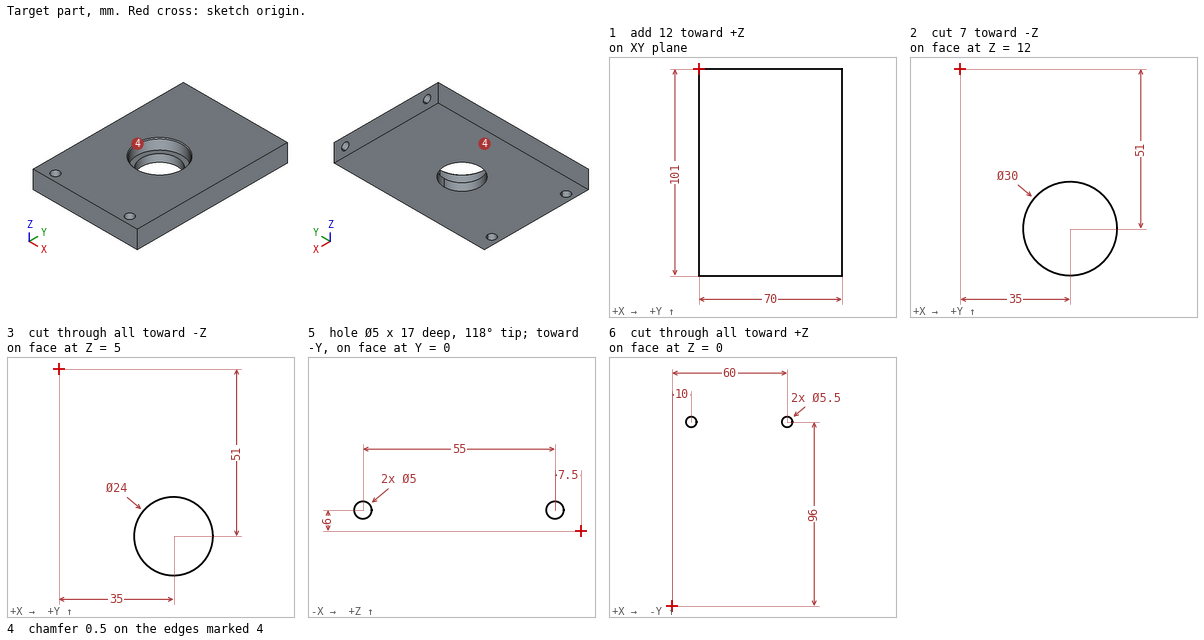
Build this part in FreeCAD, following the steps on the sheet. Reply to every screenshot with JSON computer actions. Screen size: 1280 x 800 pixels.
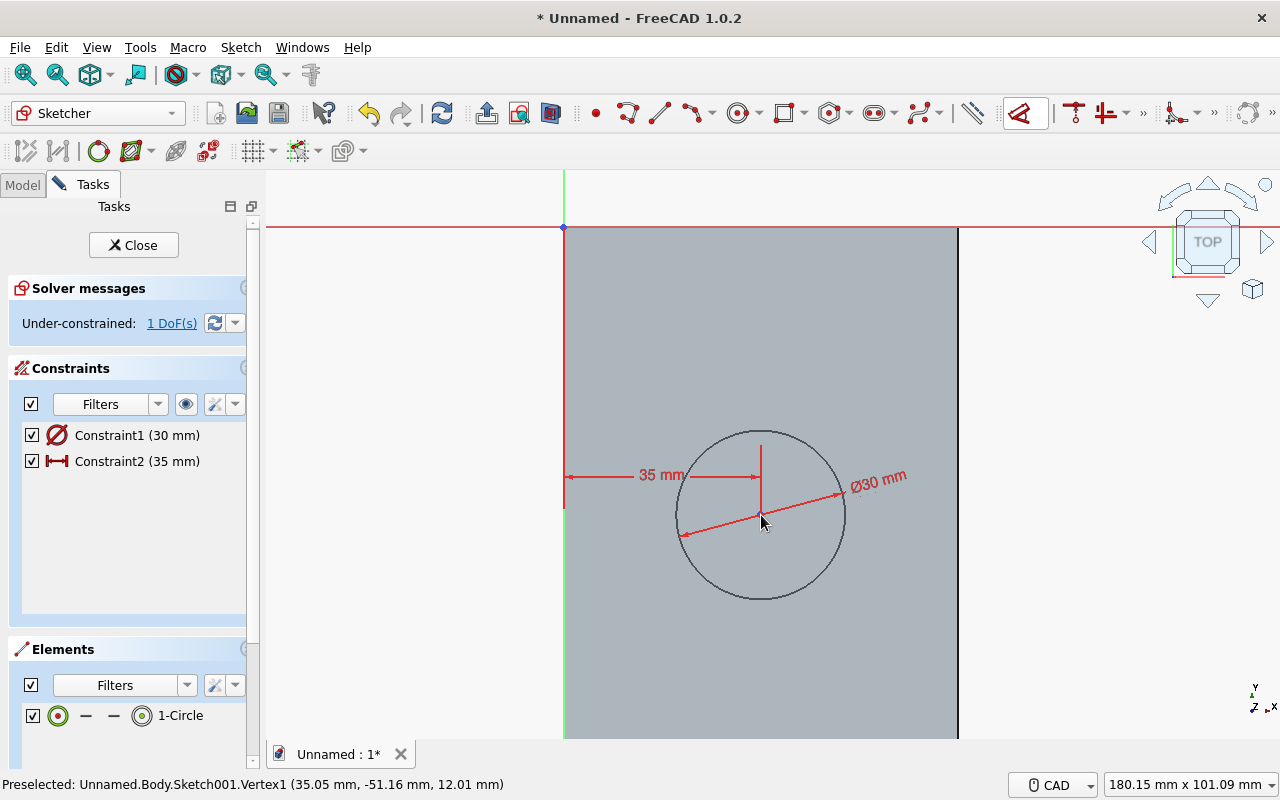
{"action": "left_click", "coordinate": [761, 515]}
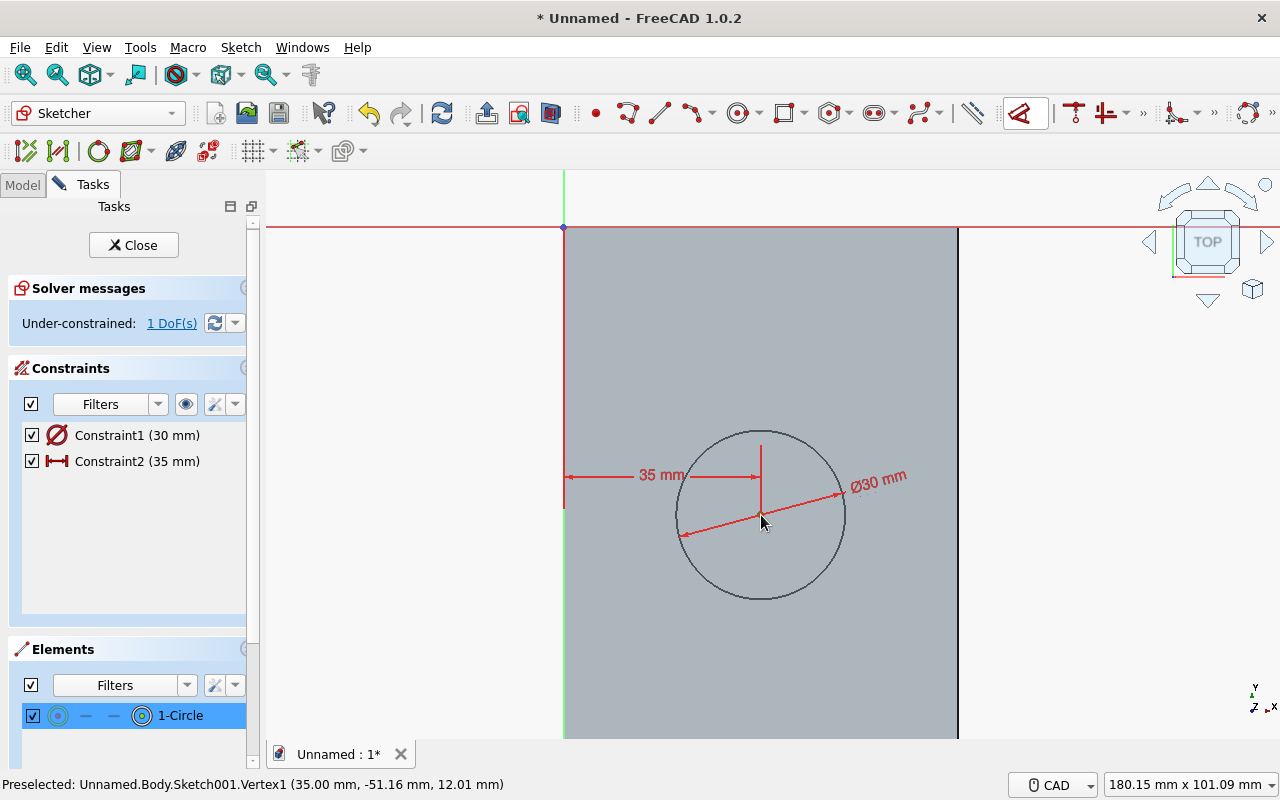
{"action": "key", "text": "i"}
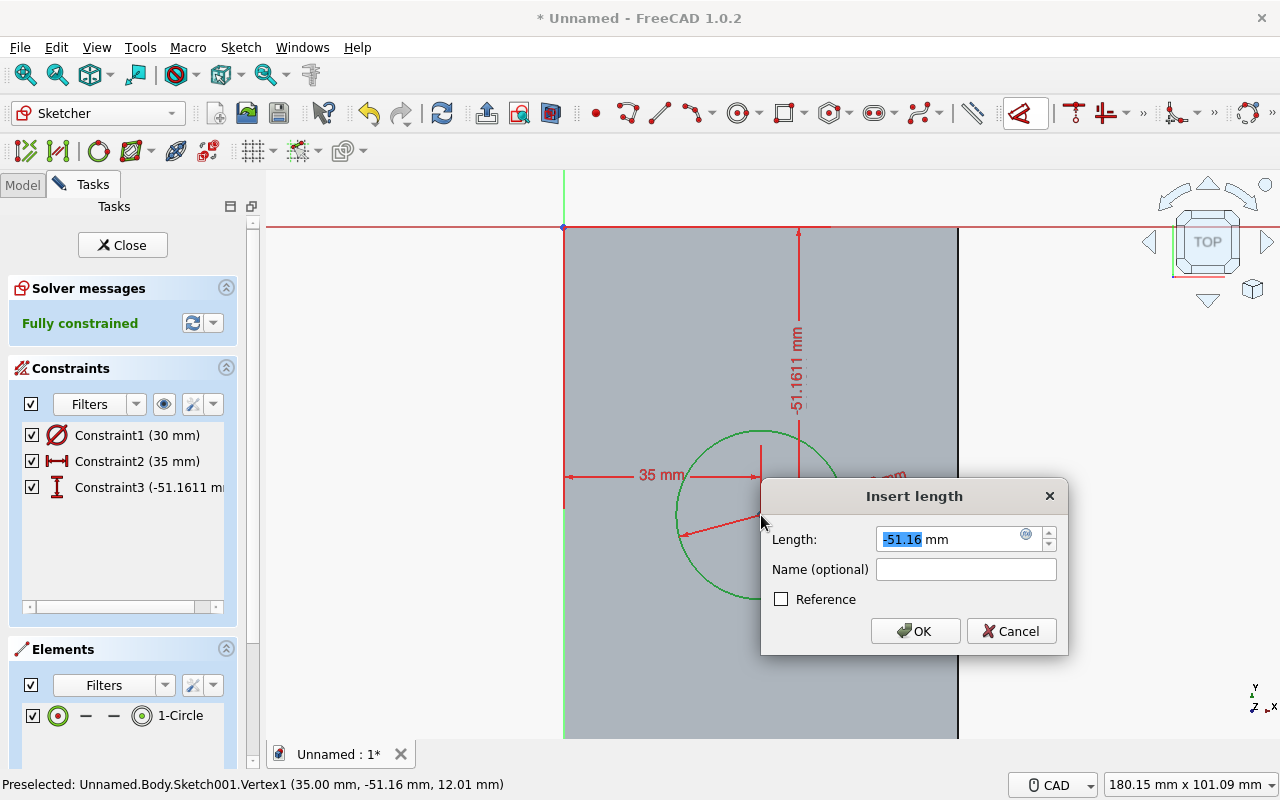
{"action": "type", "text": "-51"}
{"action": "key", "text": "Return"}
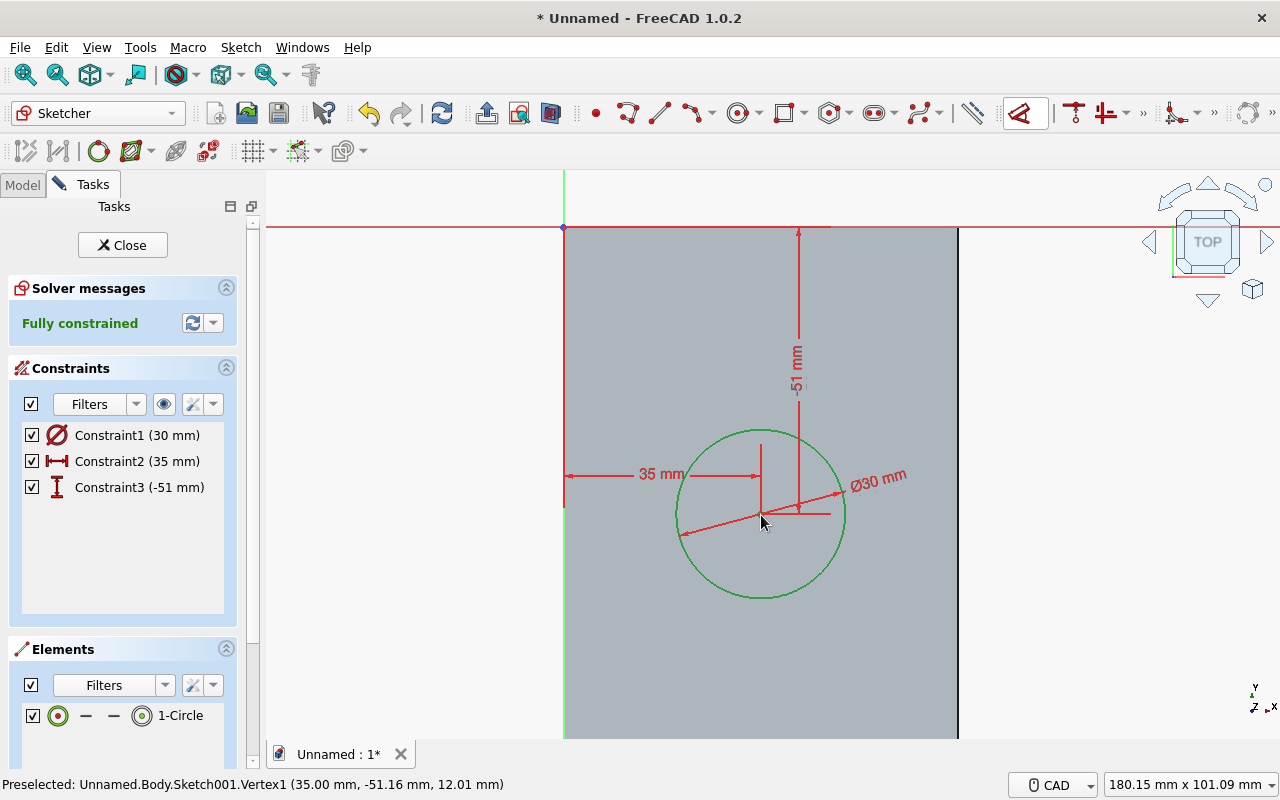
{"action": "left_click", "coordinate": [123, 245]}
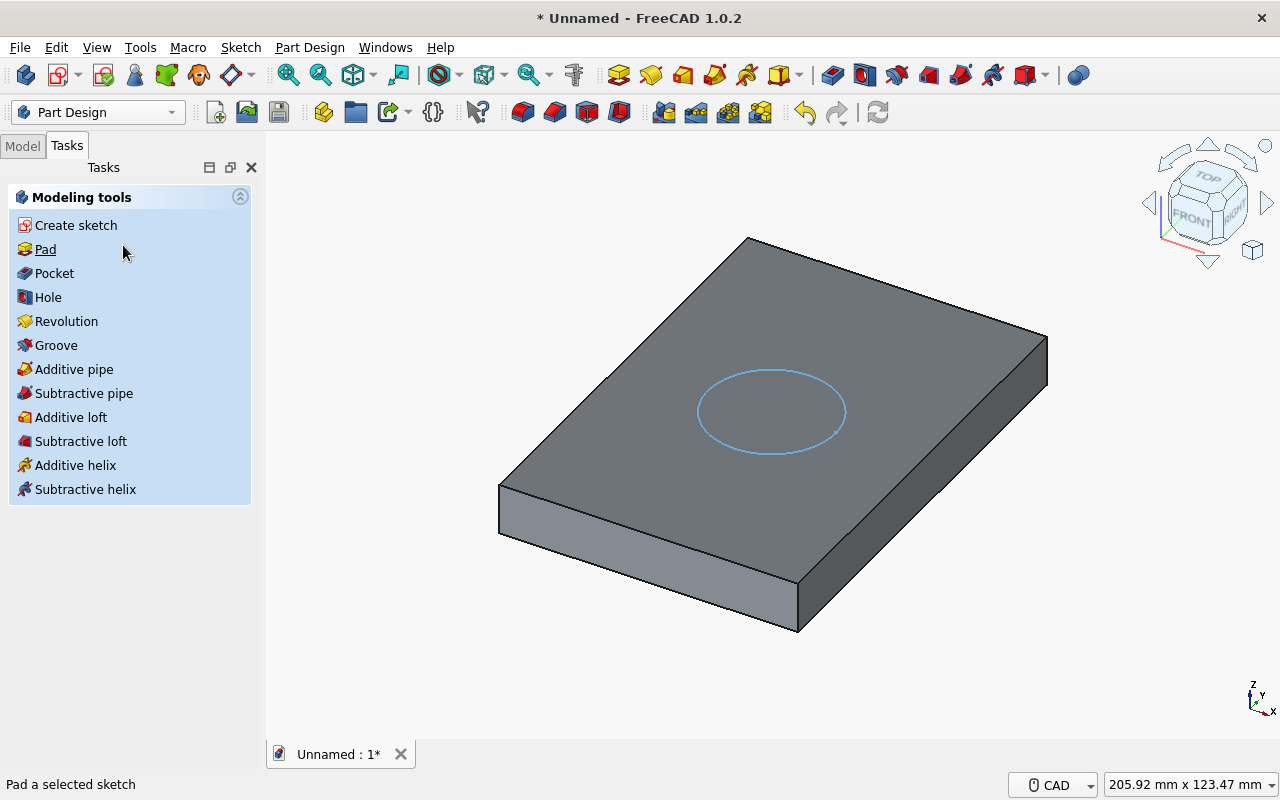
{"action": "left_click", "coordinate": [834, 76]}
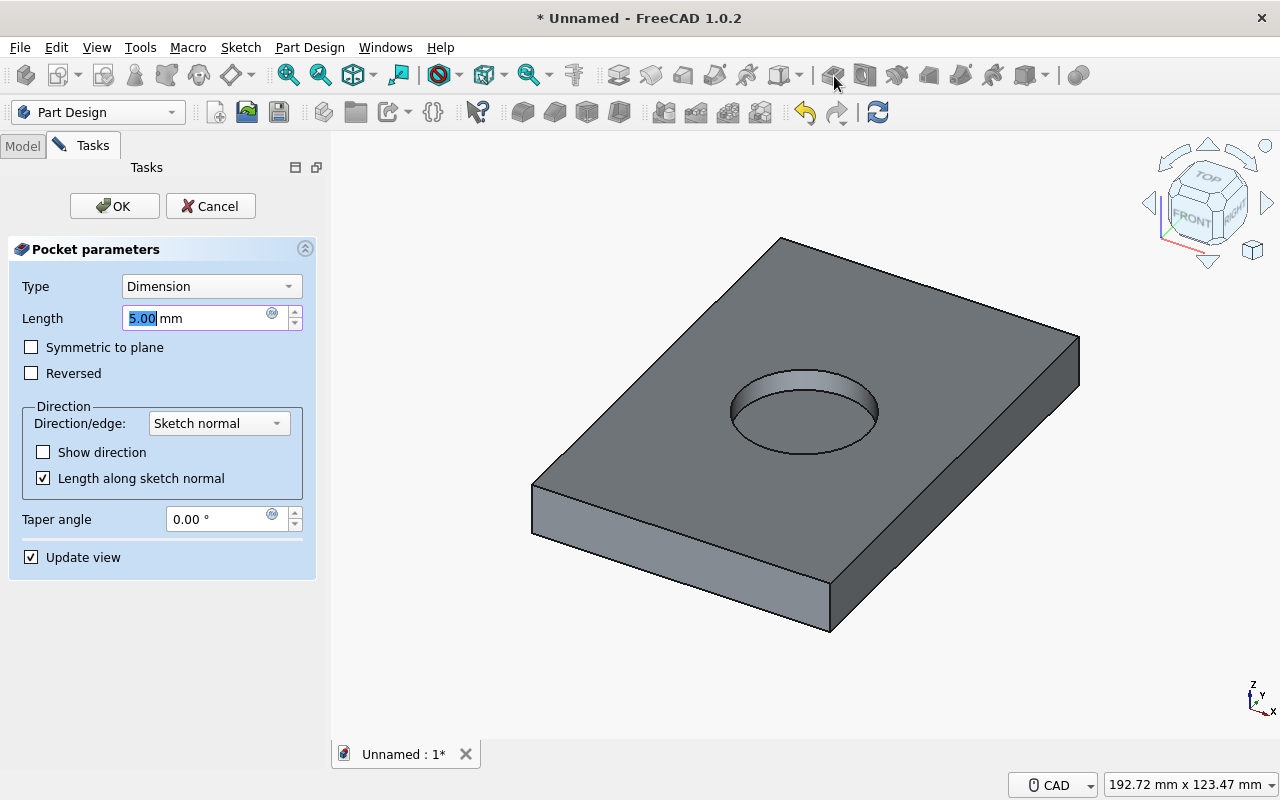
{"action": "type", "text": "7"}
{"action": "key", "text": "Tab"}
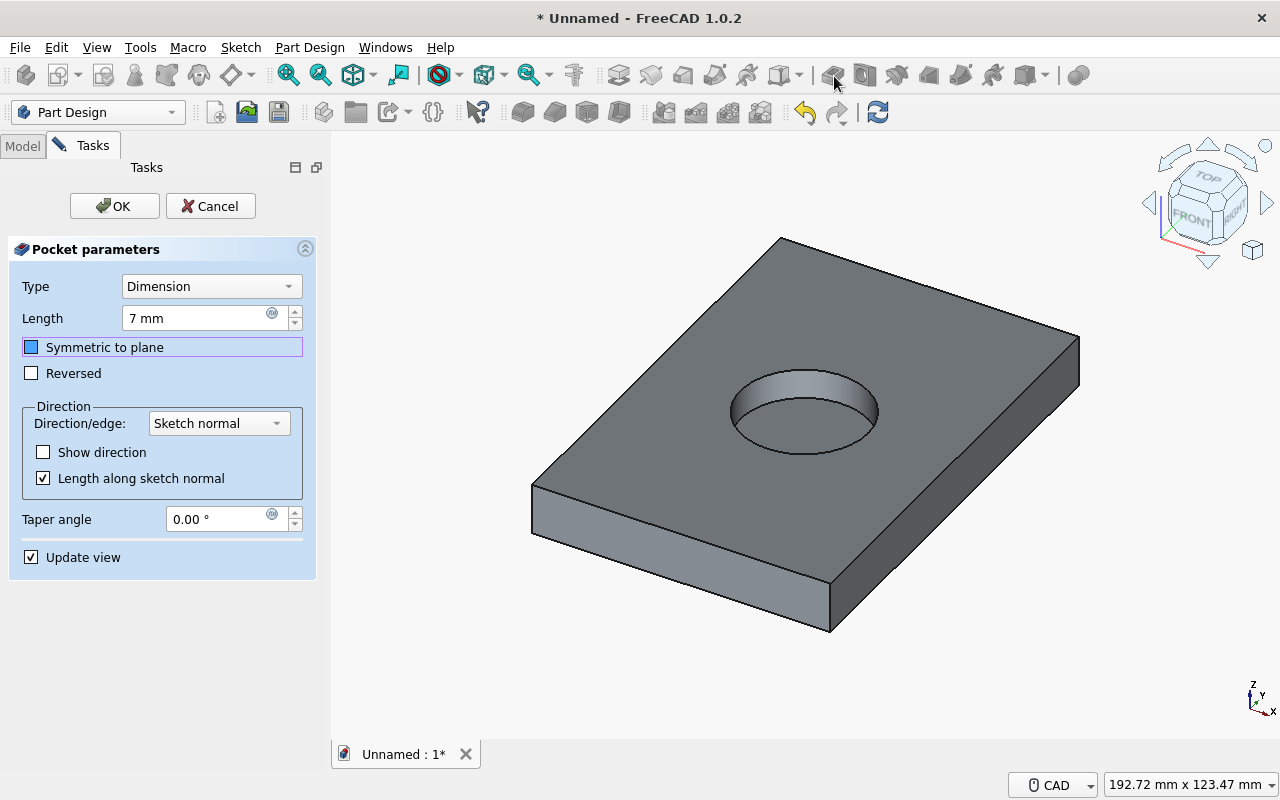
{"action": "left_click", "coordinate": [115, 206]}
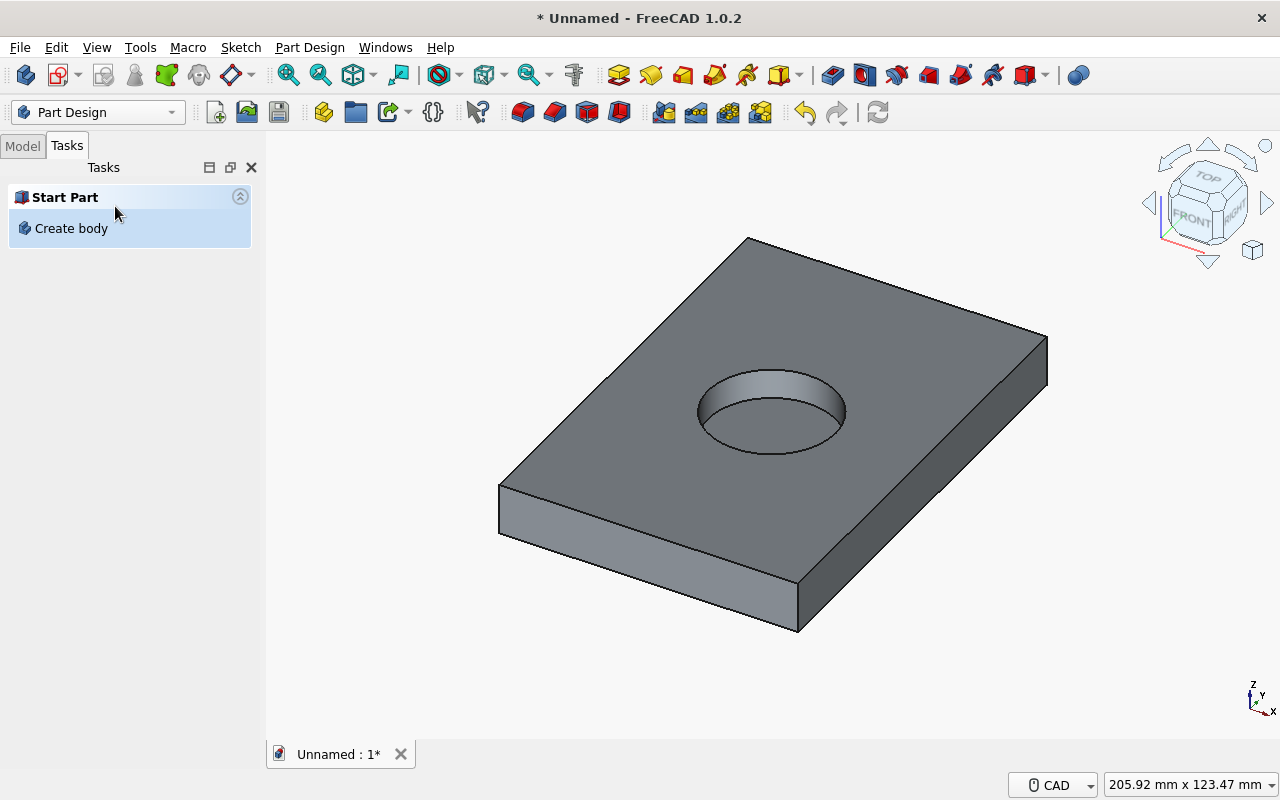
{"action": "left_click", "coordinate": [772, 439]}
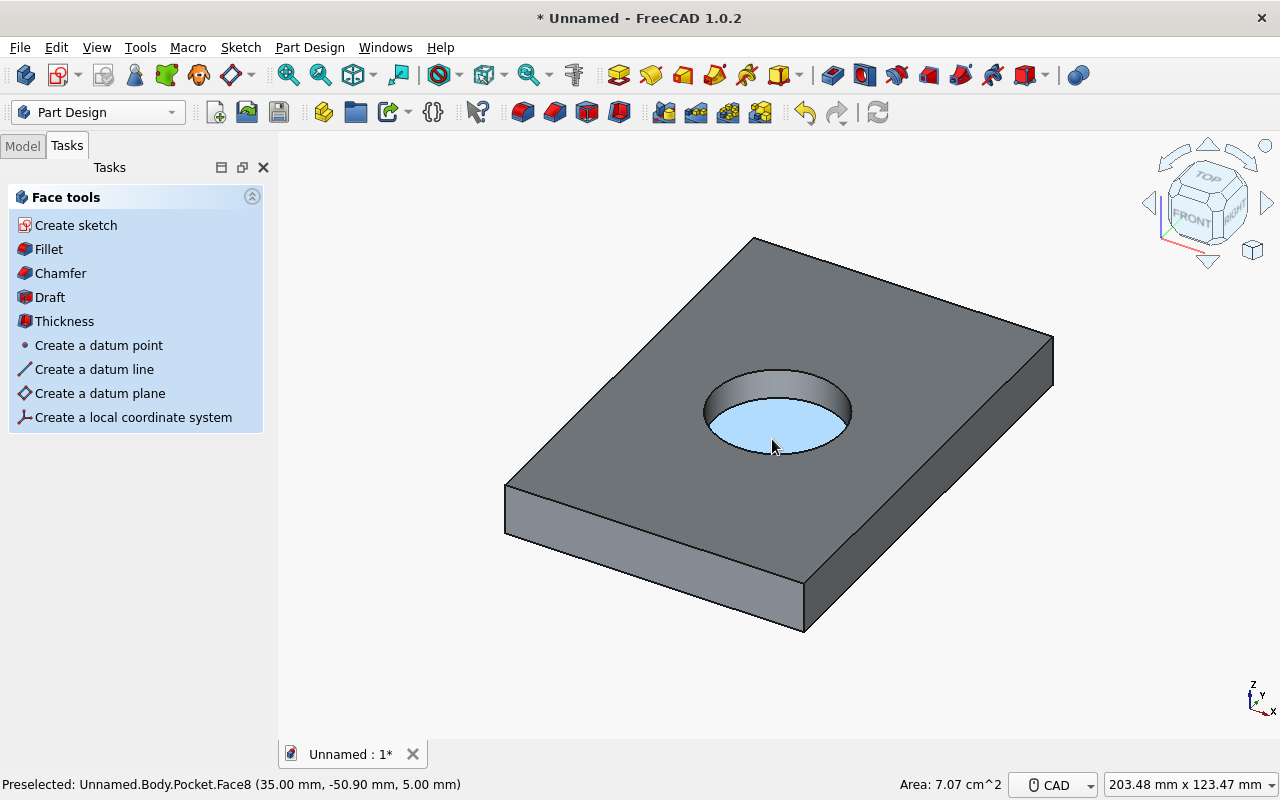
{"action": "left_click", "coordinate": [58, 76]}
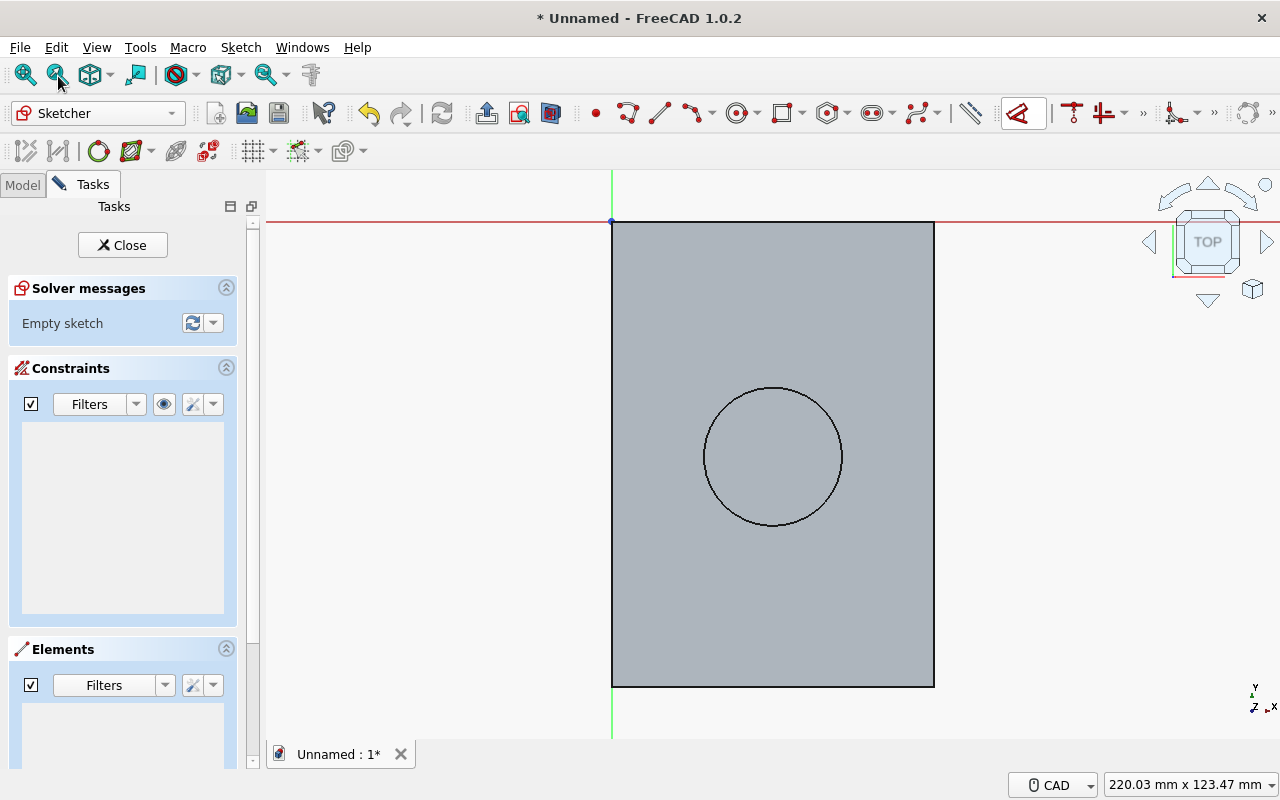
{"action": "left_click", "coordinate": [552, 114]}